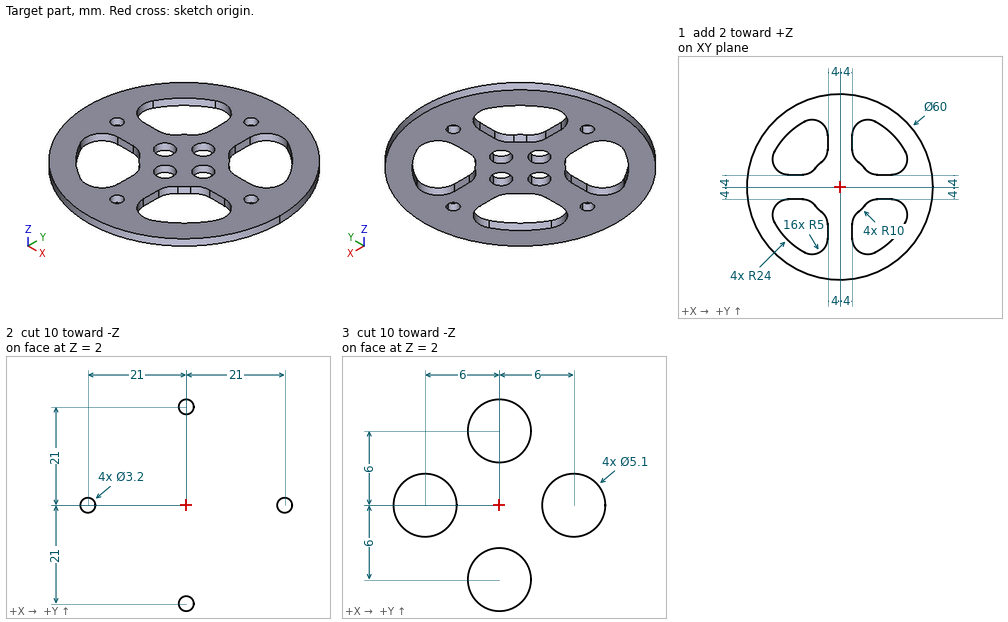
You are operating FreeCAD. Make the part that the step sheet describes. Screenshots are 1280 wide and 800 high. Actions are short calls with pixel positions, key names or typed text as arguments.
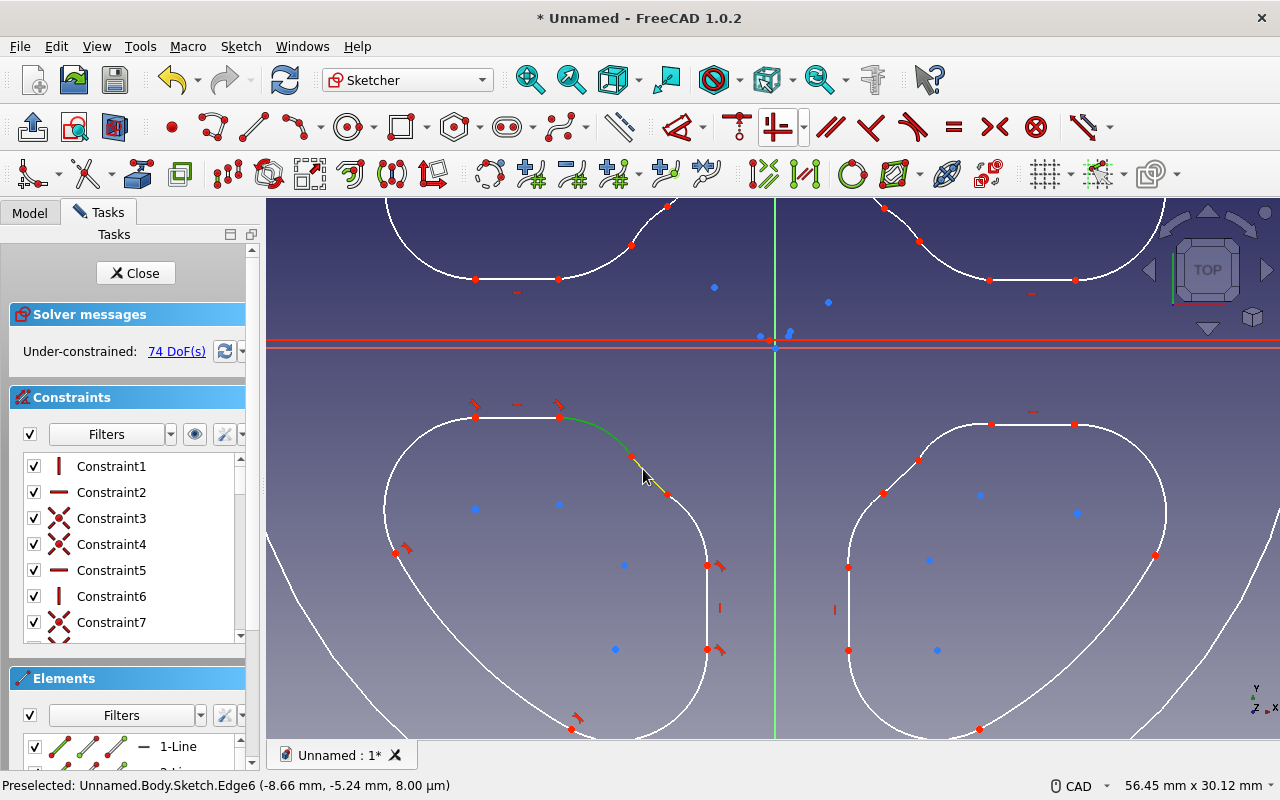
click(642, 469)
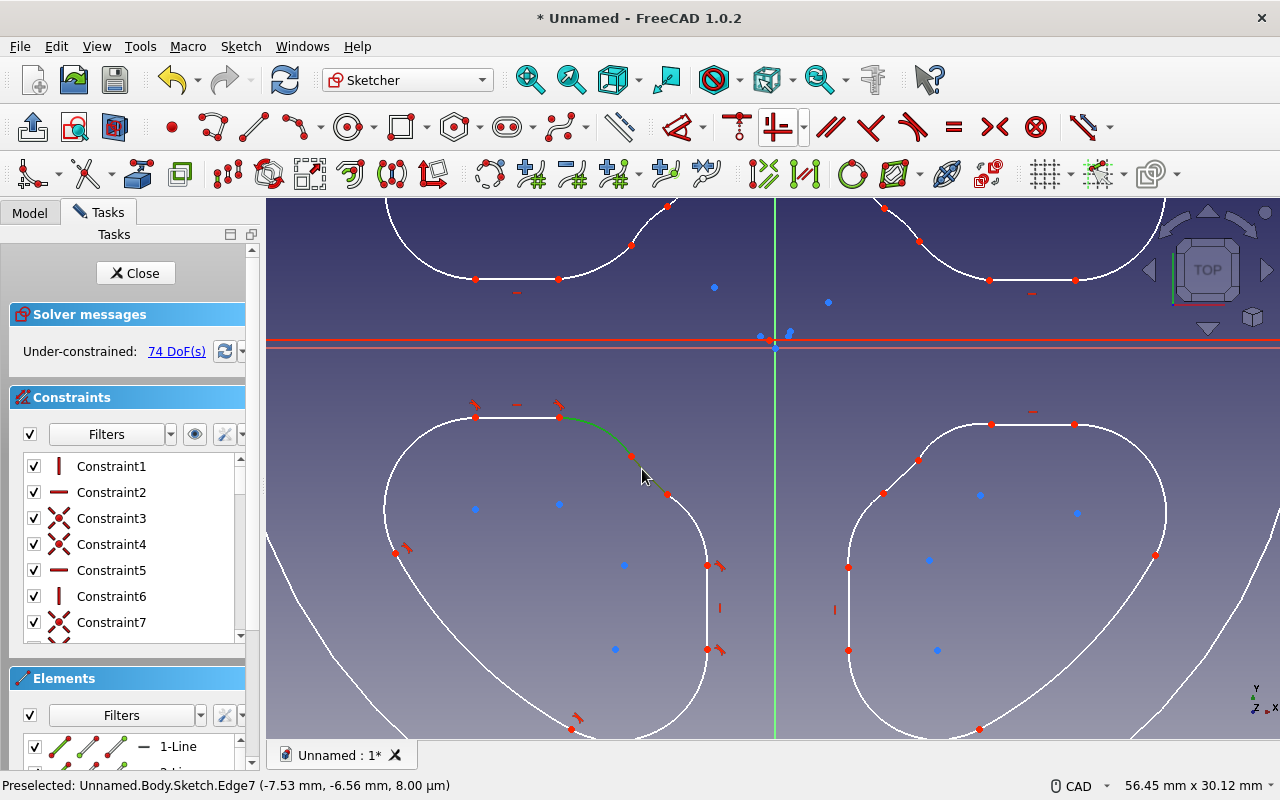
click(913, 128)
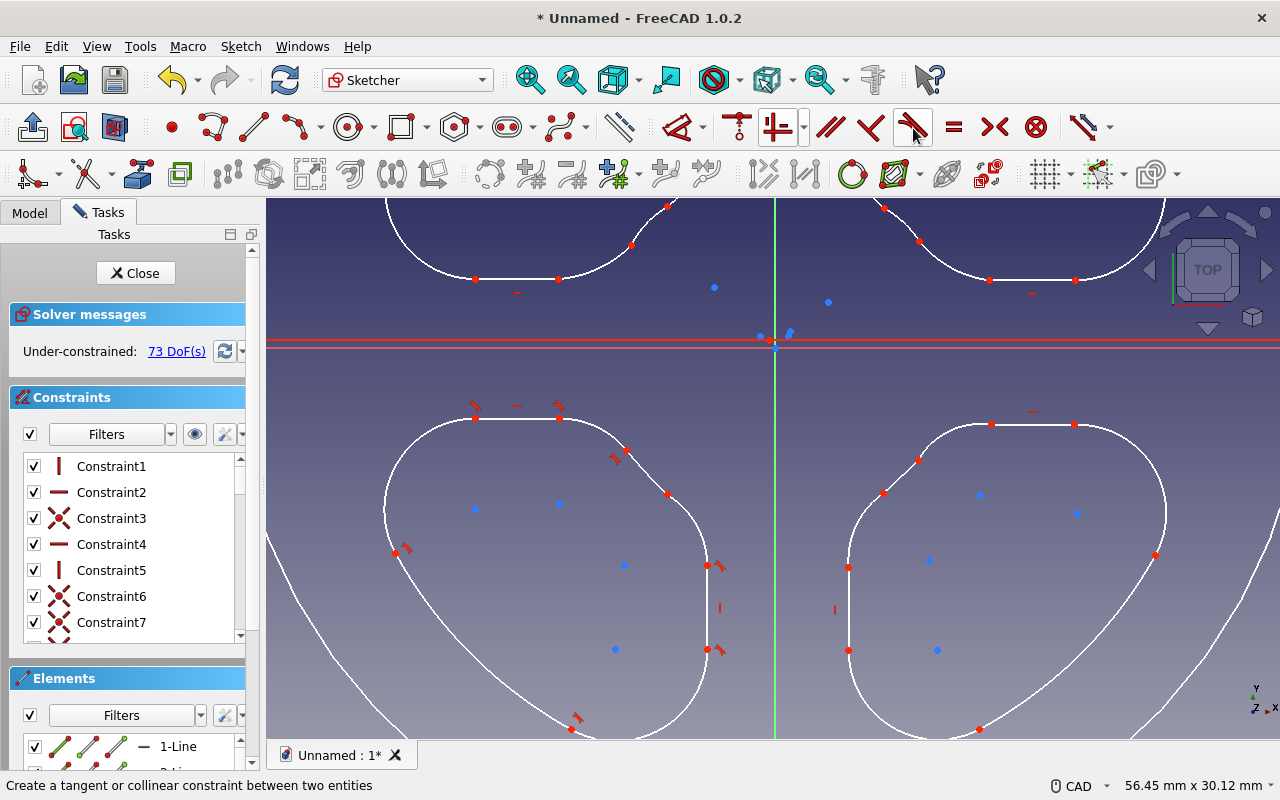
click(638, 464)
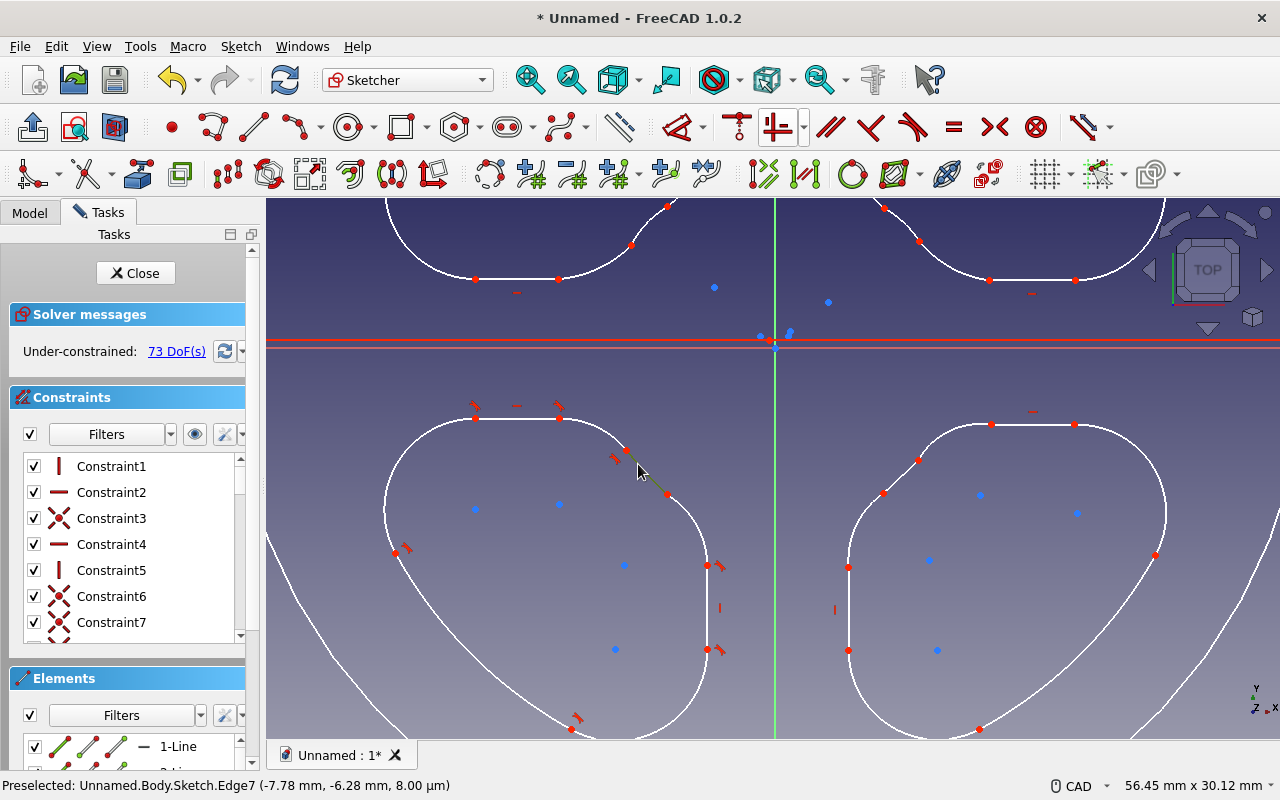
click(703, 541)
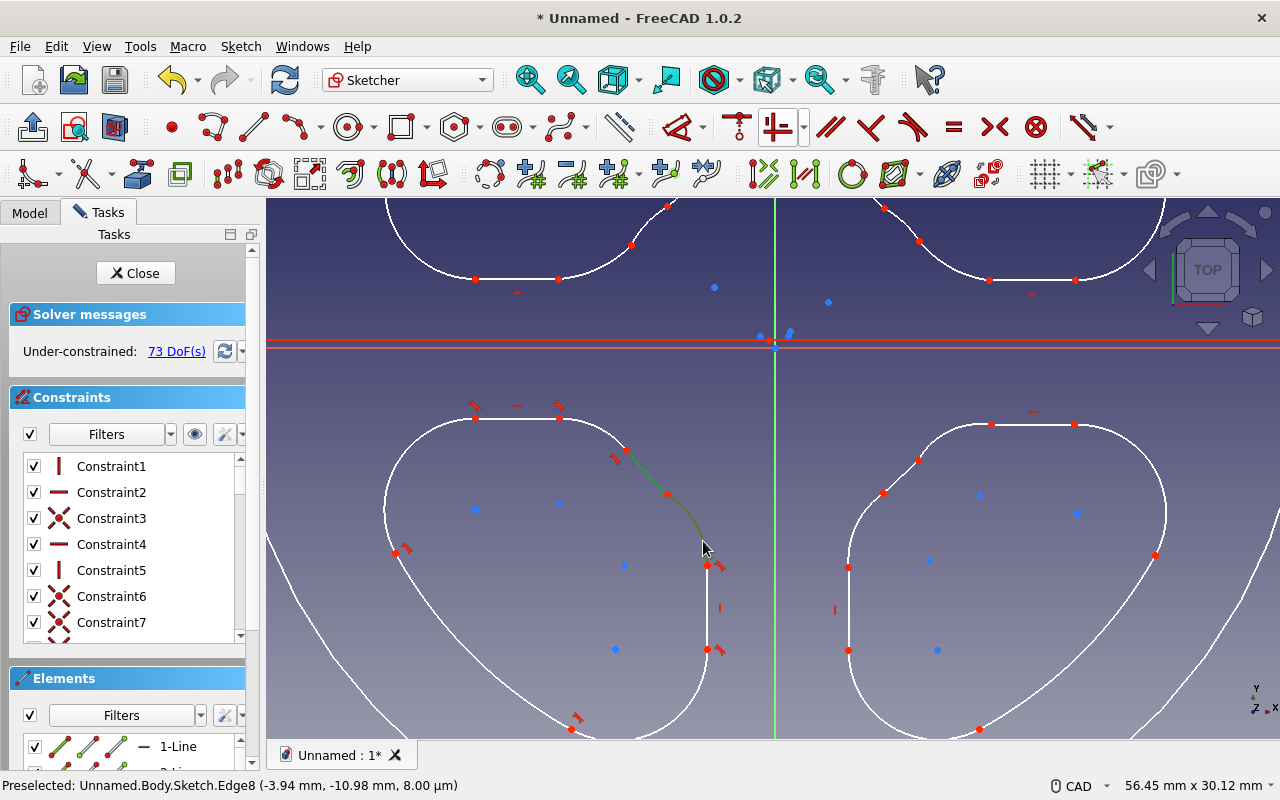
click(913, 128)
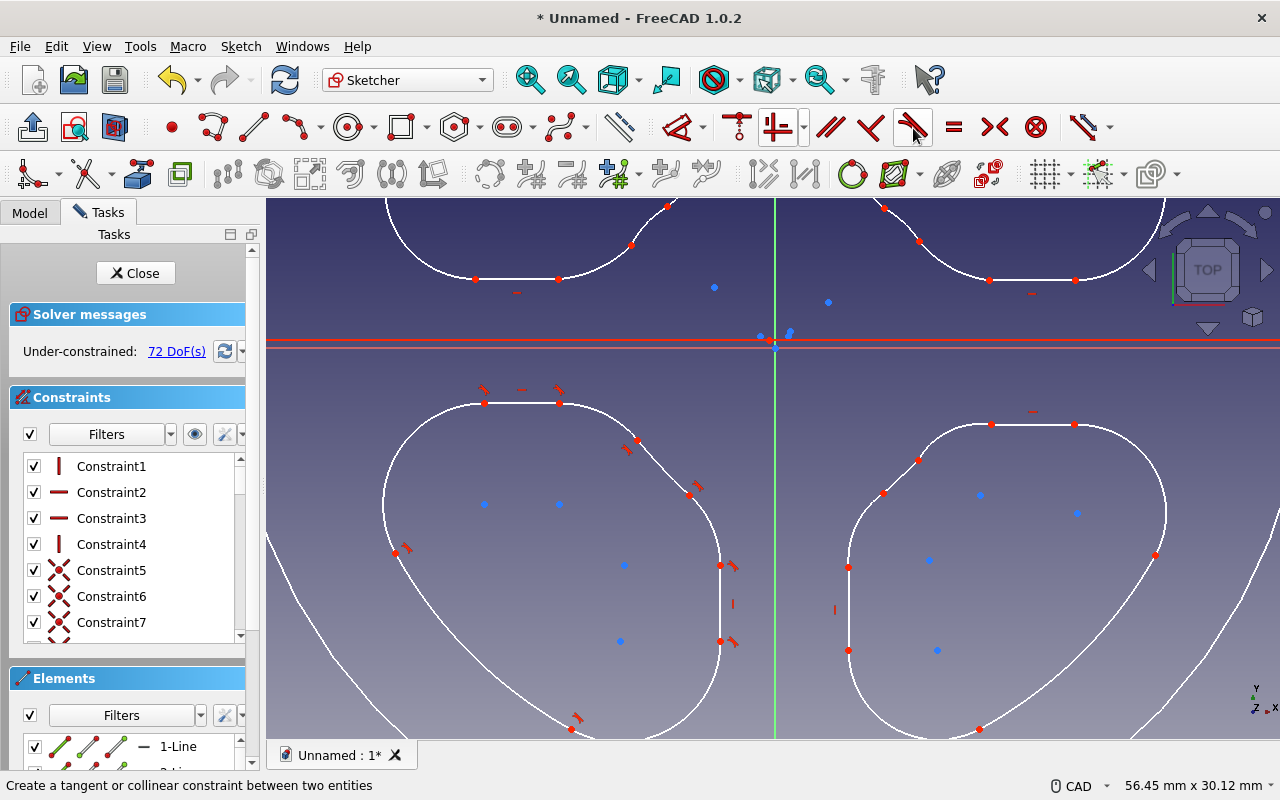
click(1016, 425)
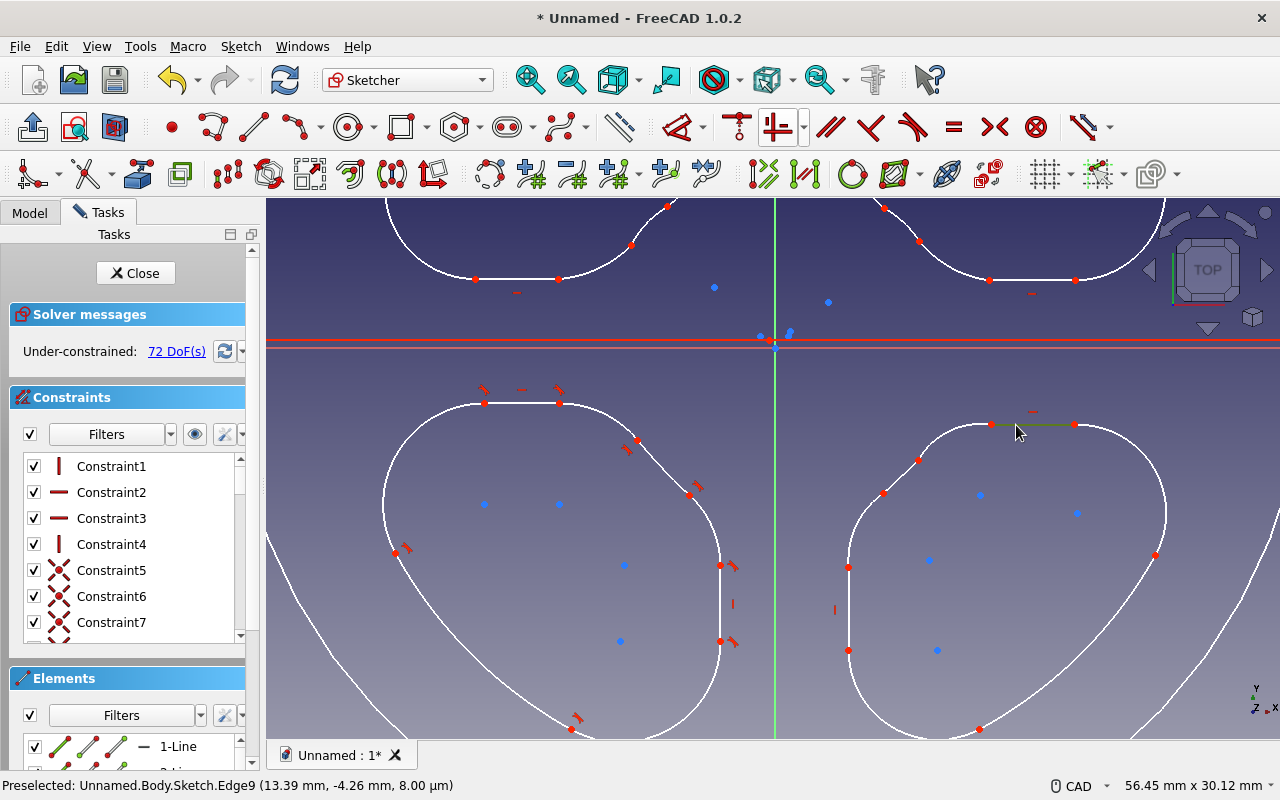
click(1111, 431)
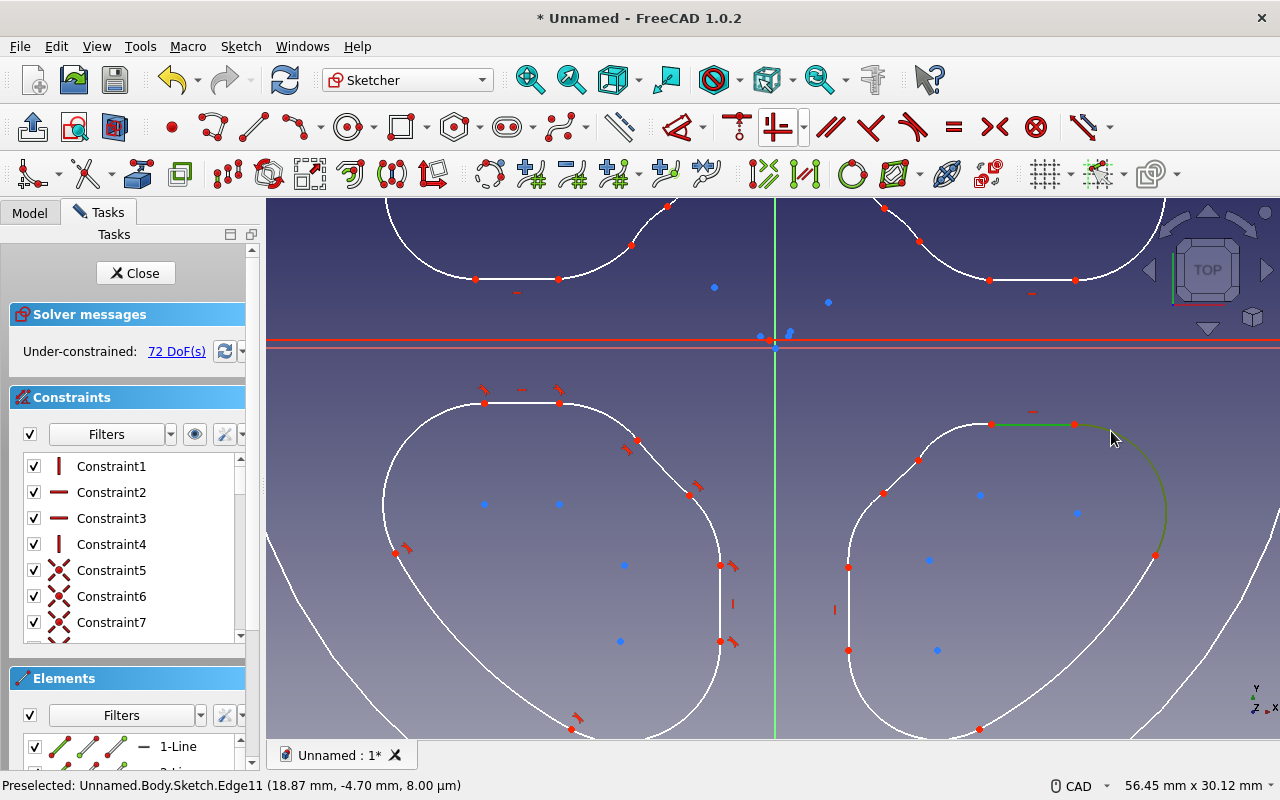
click(913, 128)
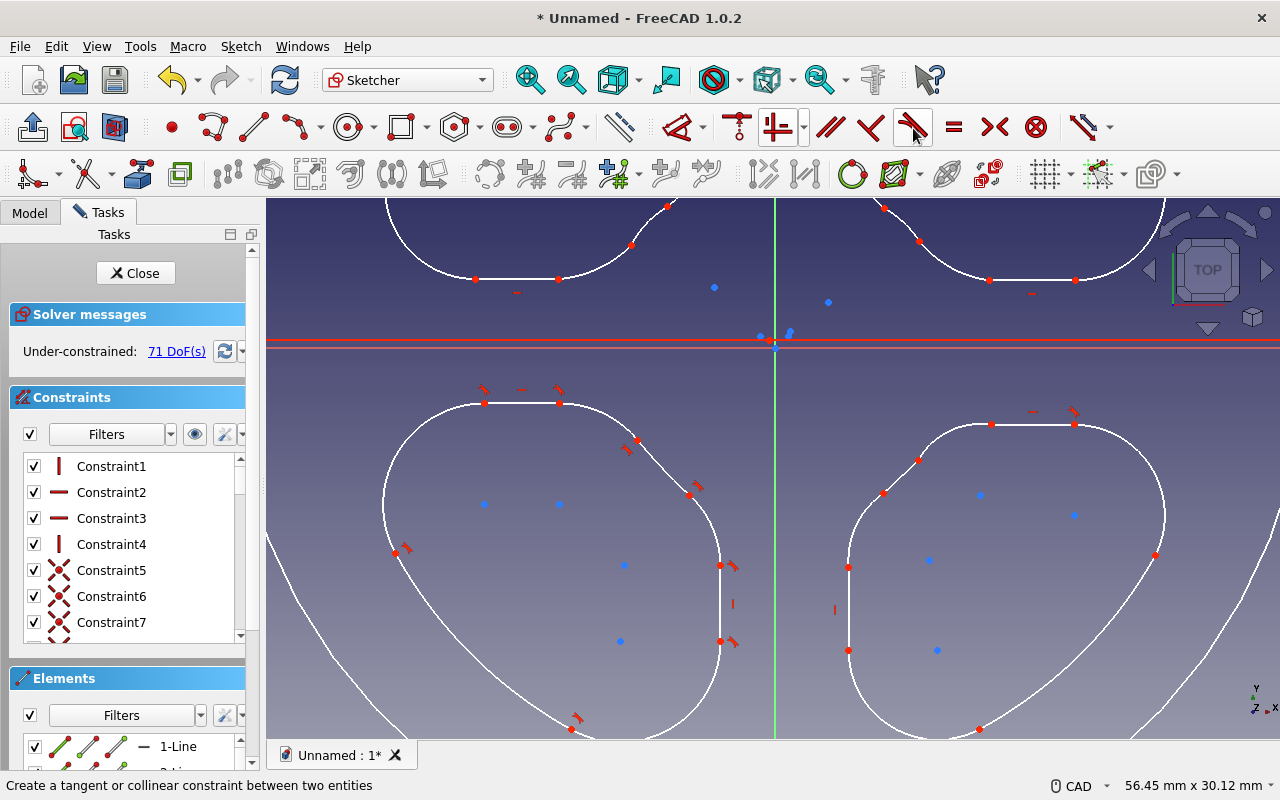
click(1016, 425)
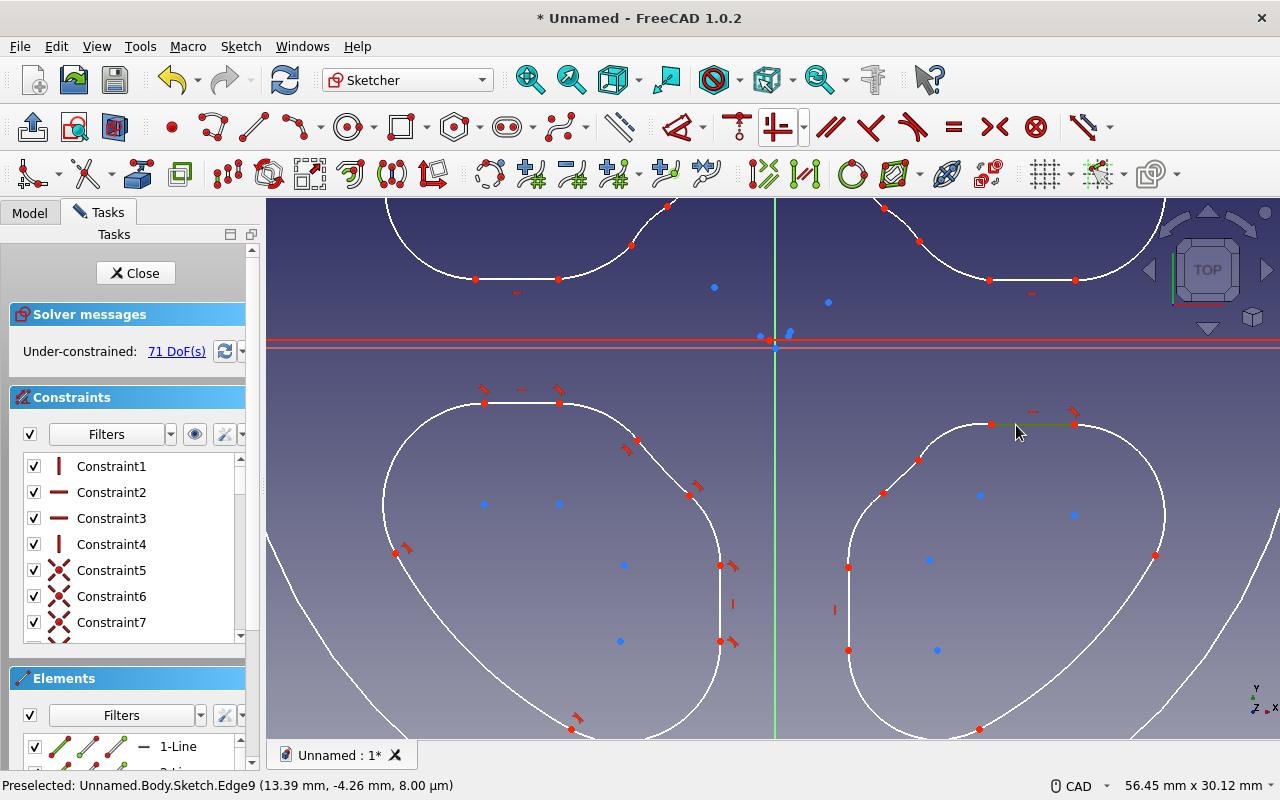
click(966, 426)